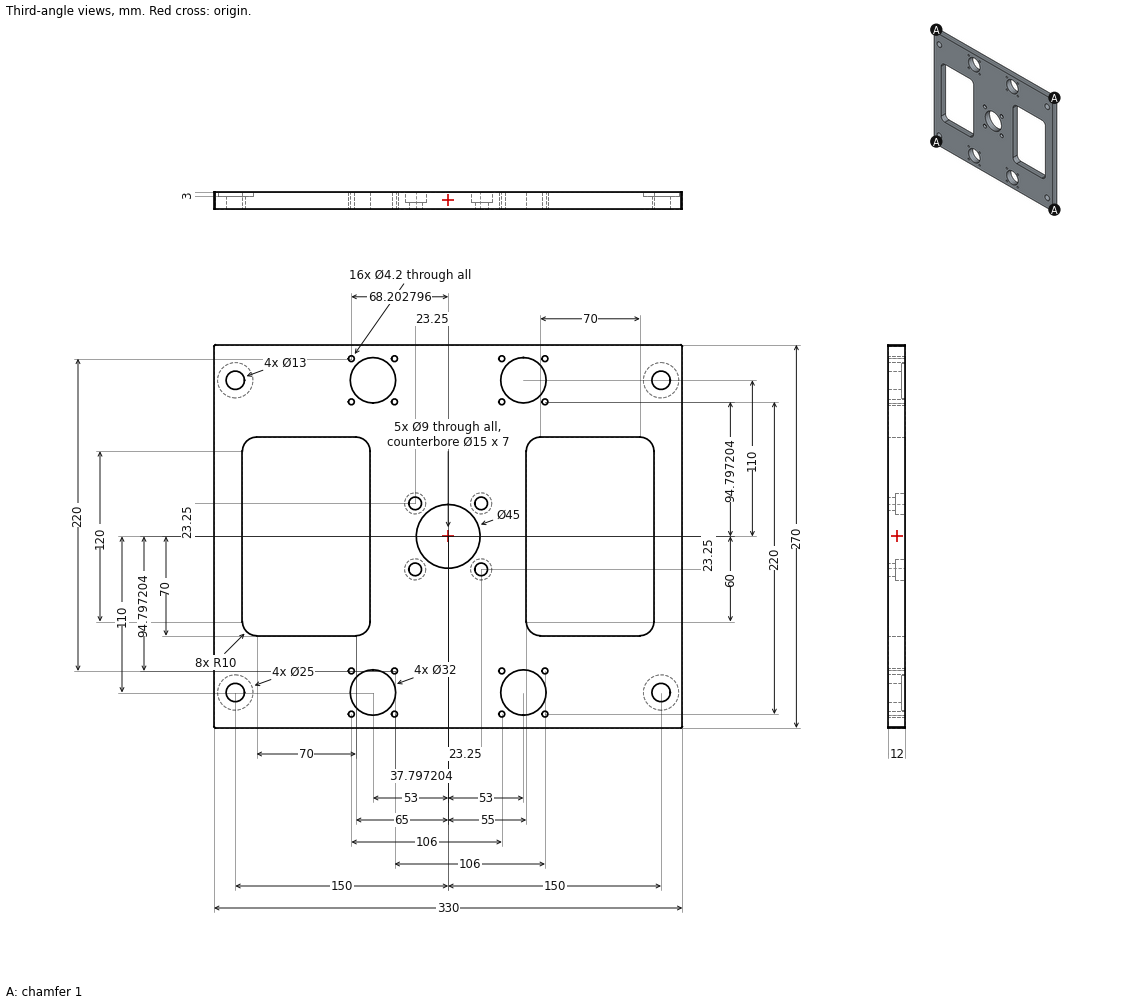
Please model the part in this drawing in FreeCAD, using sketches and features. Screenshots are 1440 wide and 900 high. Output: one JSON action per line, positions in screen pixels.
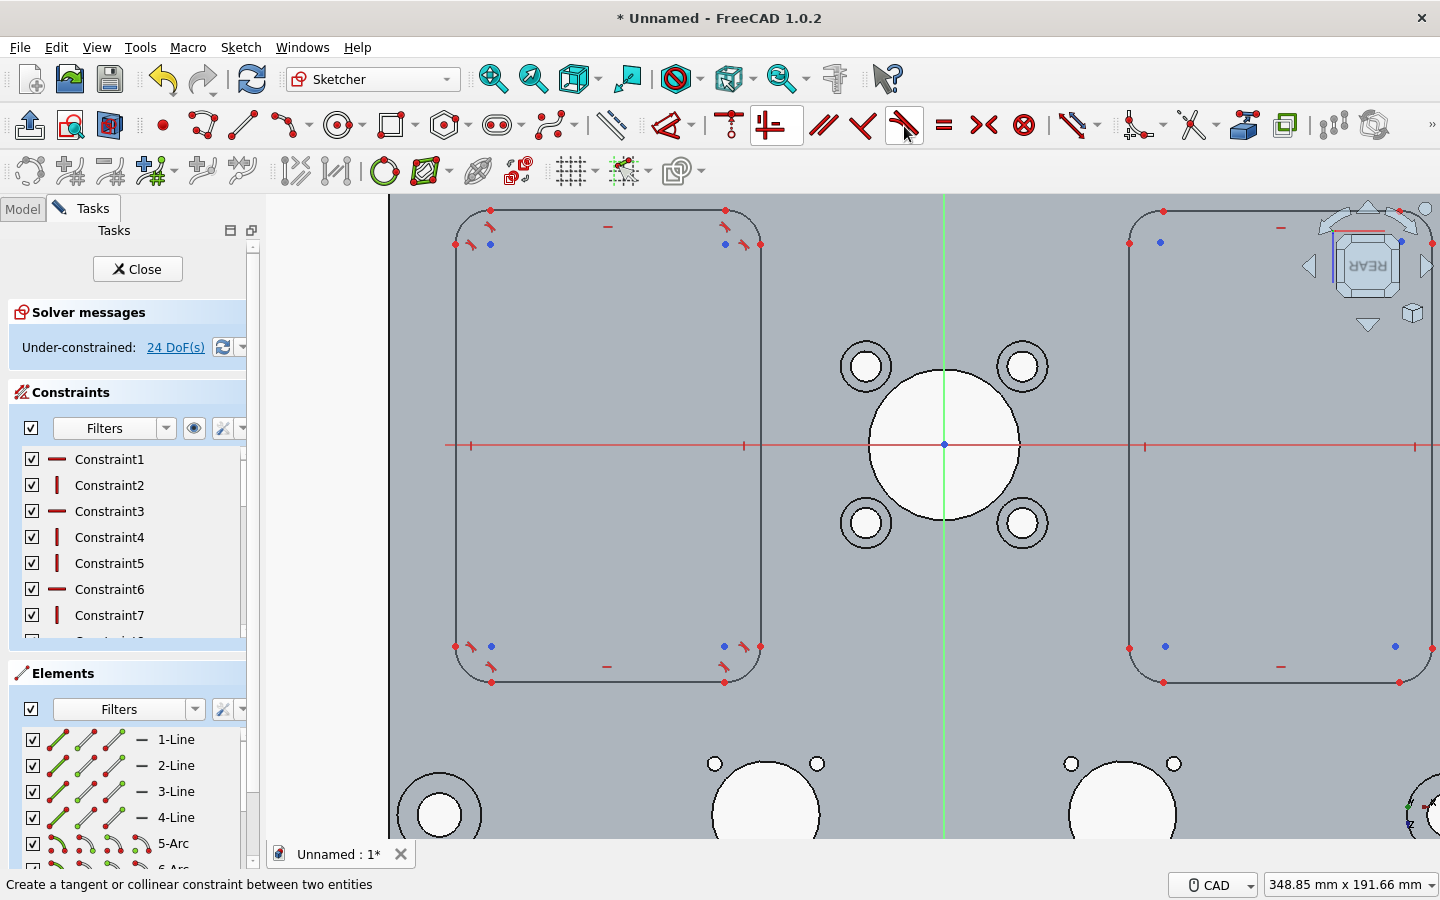
{"action": "left_click", "coordinate": [1129, 365]}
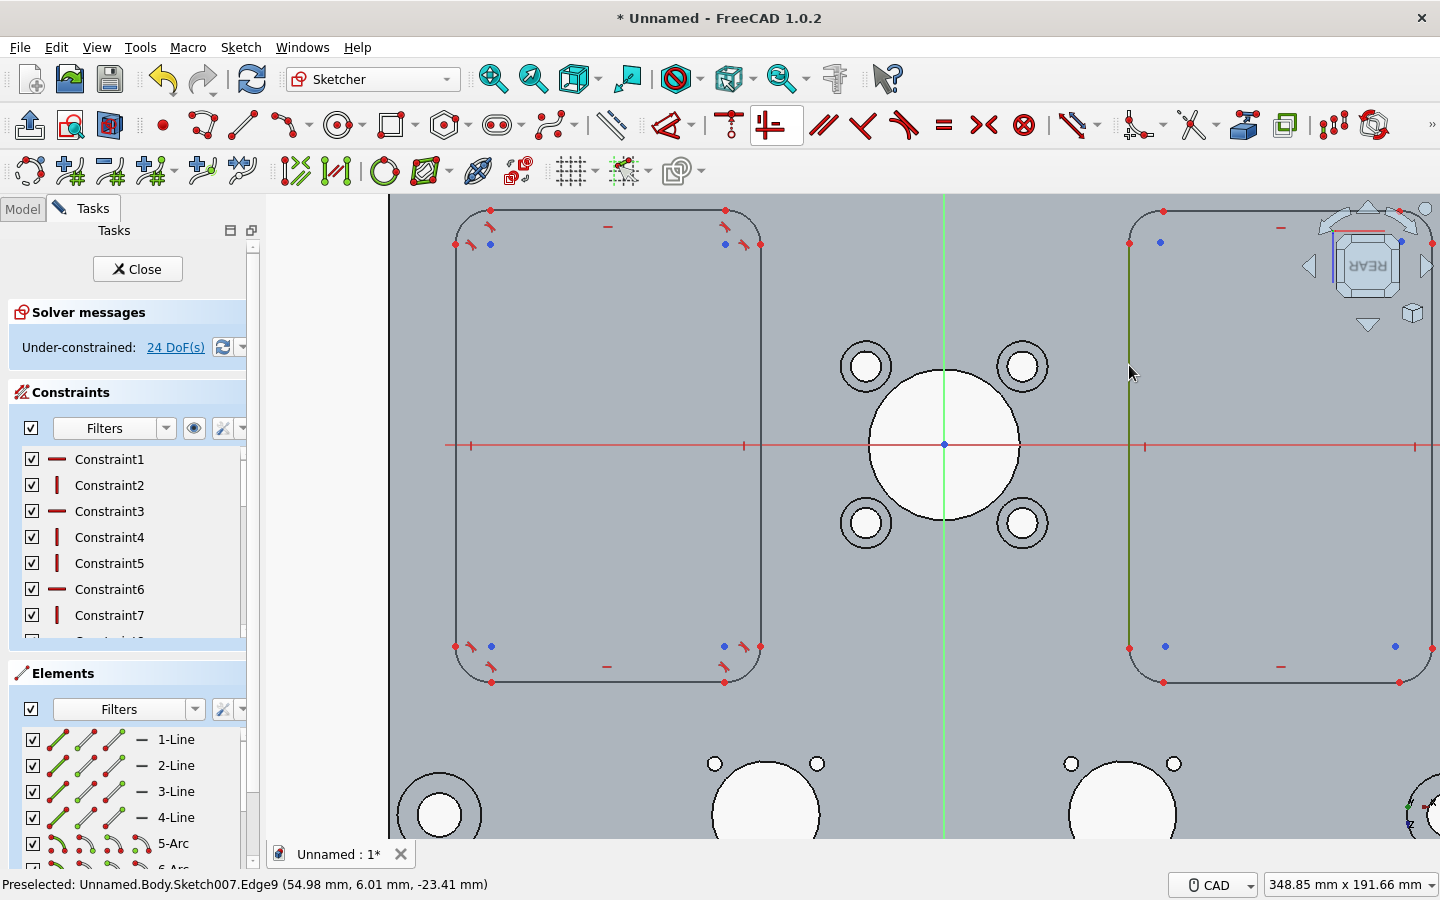
{"action": "left_click", "coordinate": [1133, 663]}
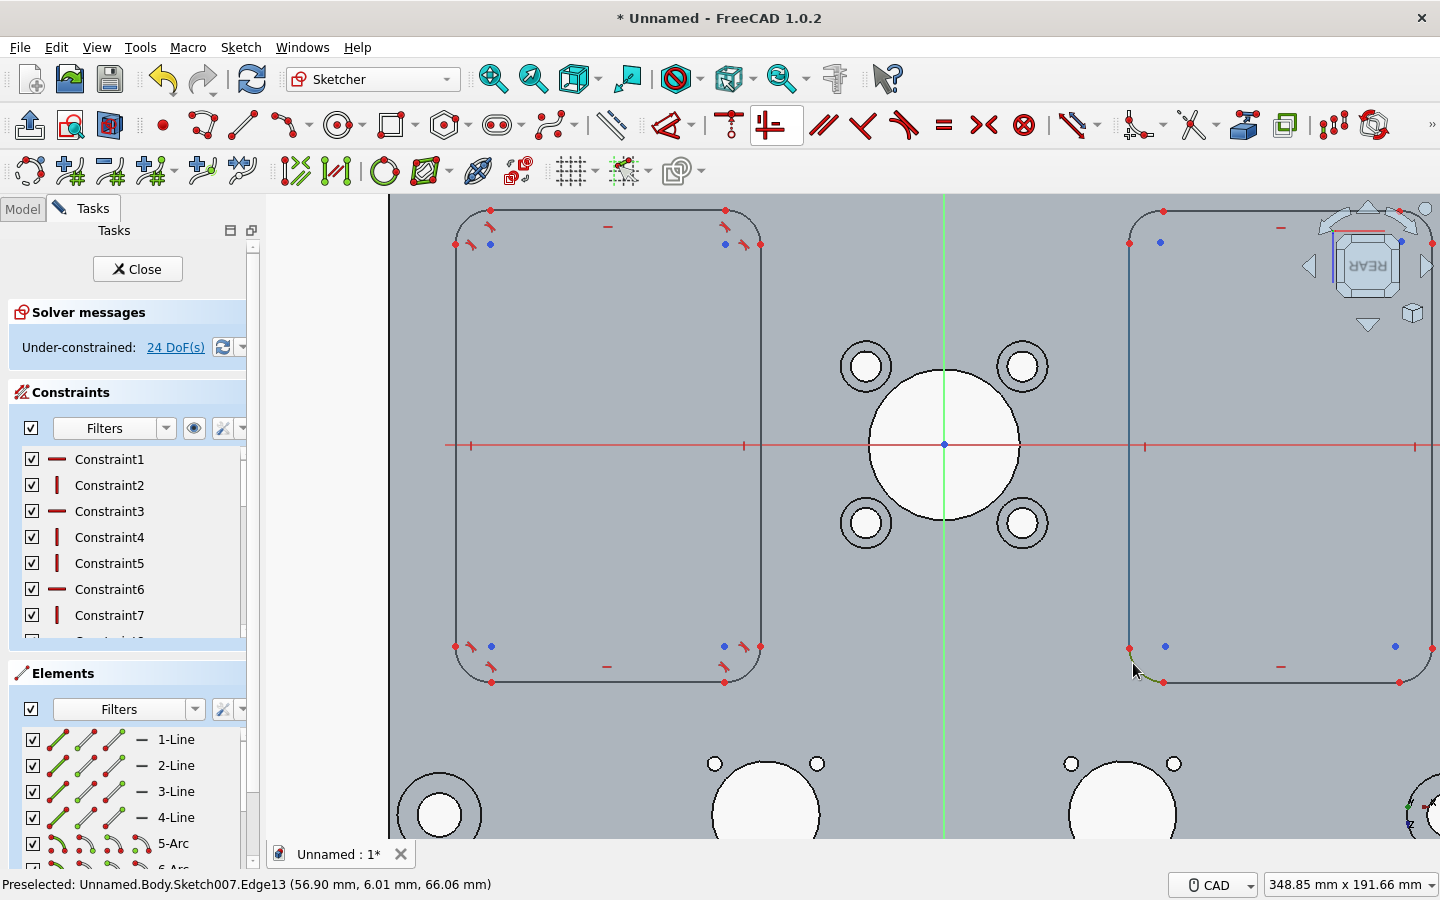
{"action": "left_click", "coordinate": [904, 126]}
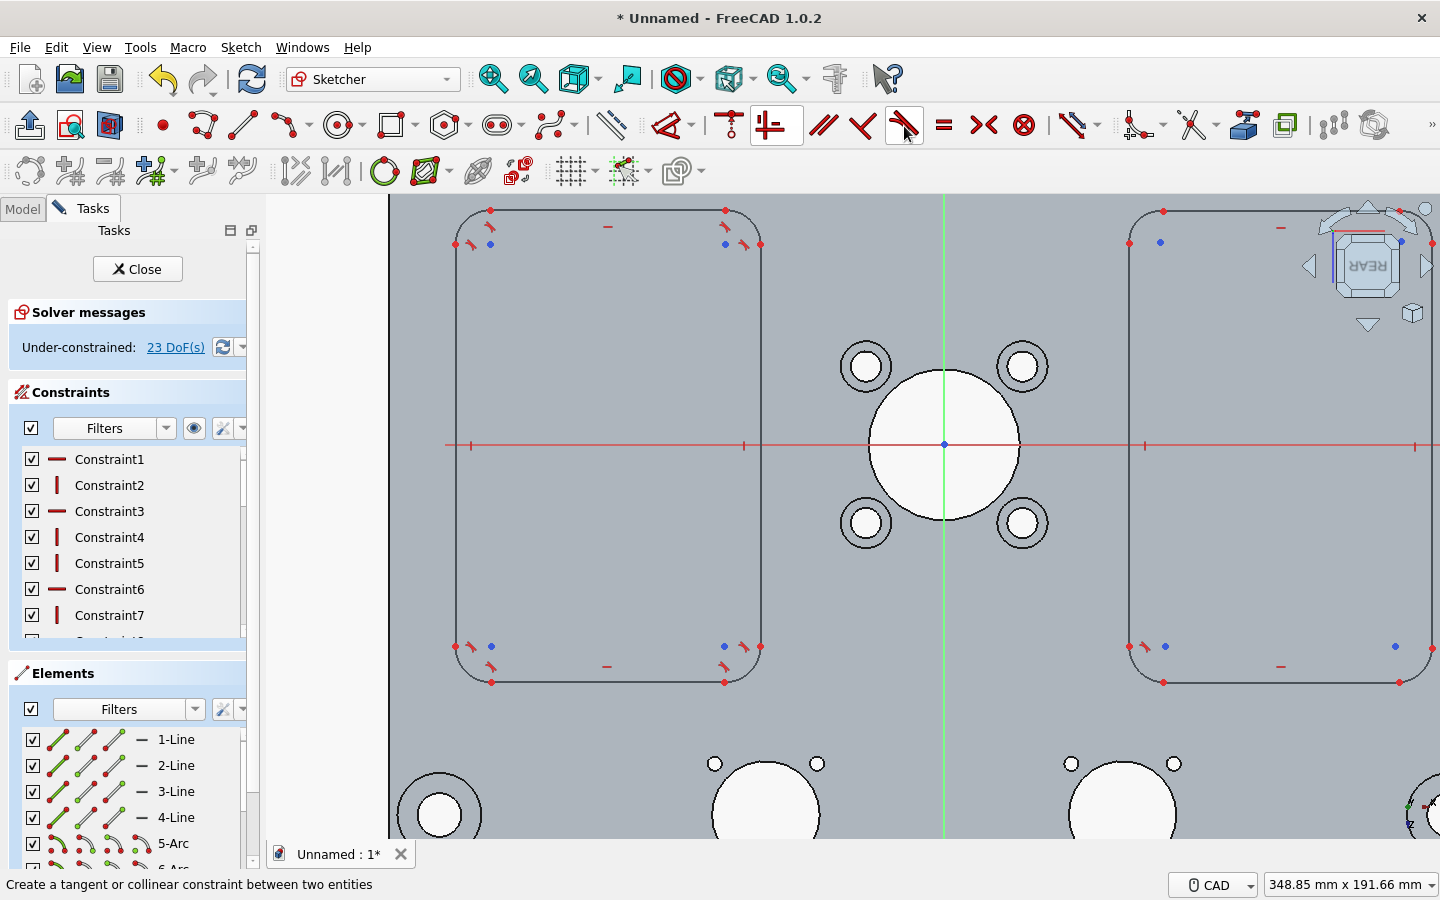
{"action": "left_click", "coordinate": [1129, 365]}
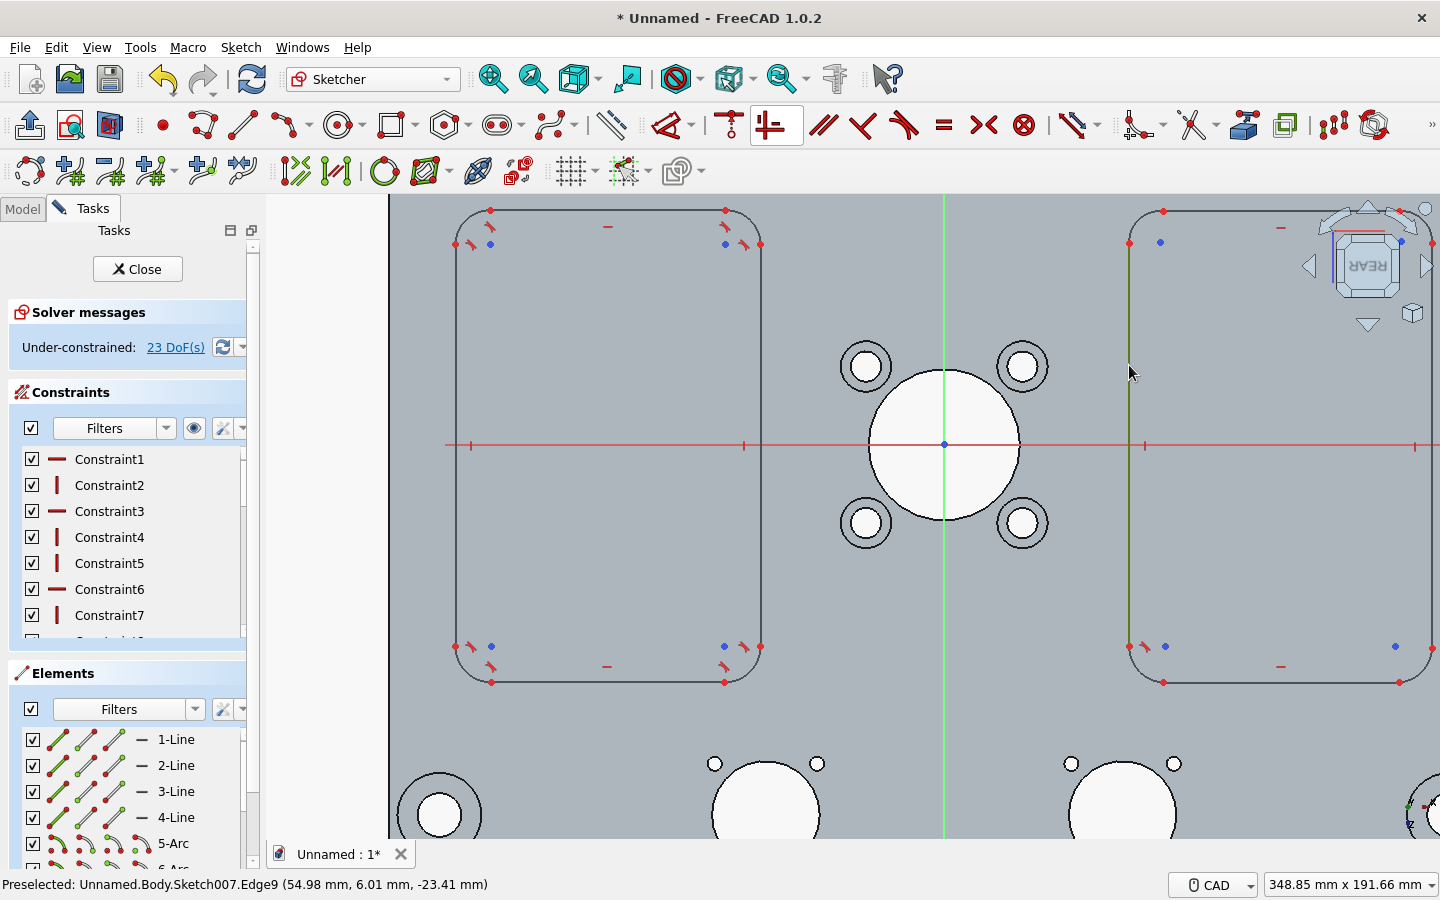
{"action": "left_click", "coordinate": [1132, 228]}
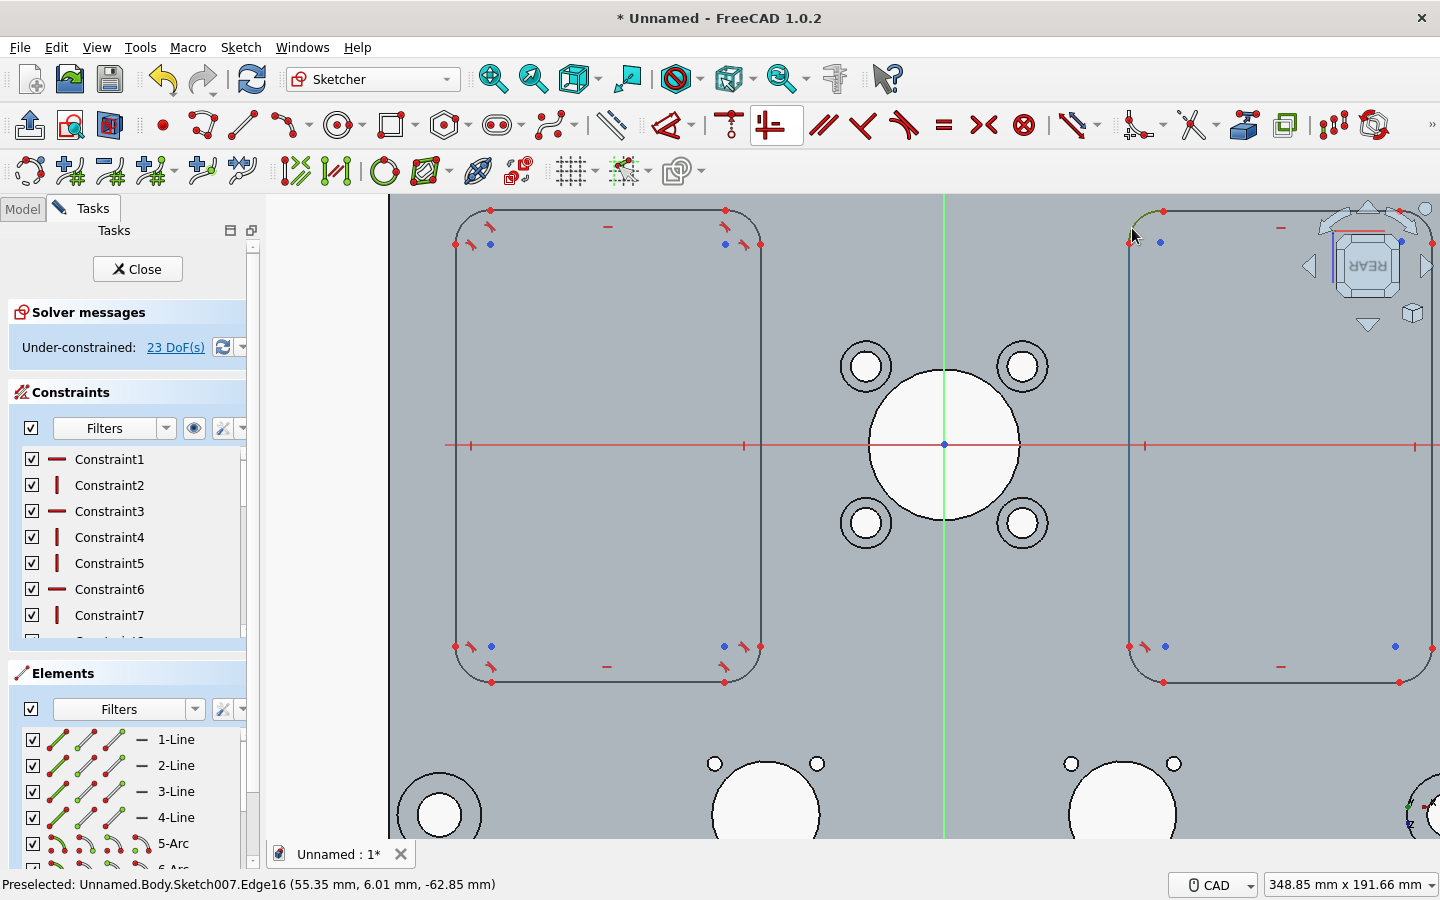
{"action": "left_click", "coordinate": [904, 126]}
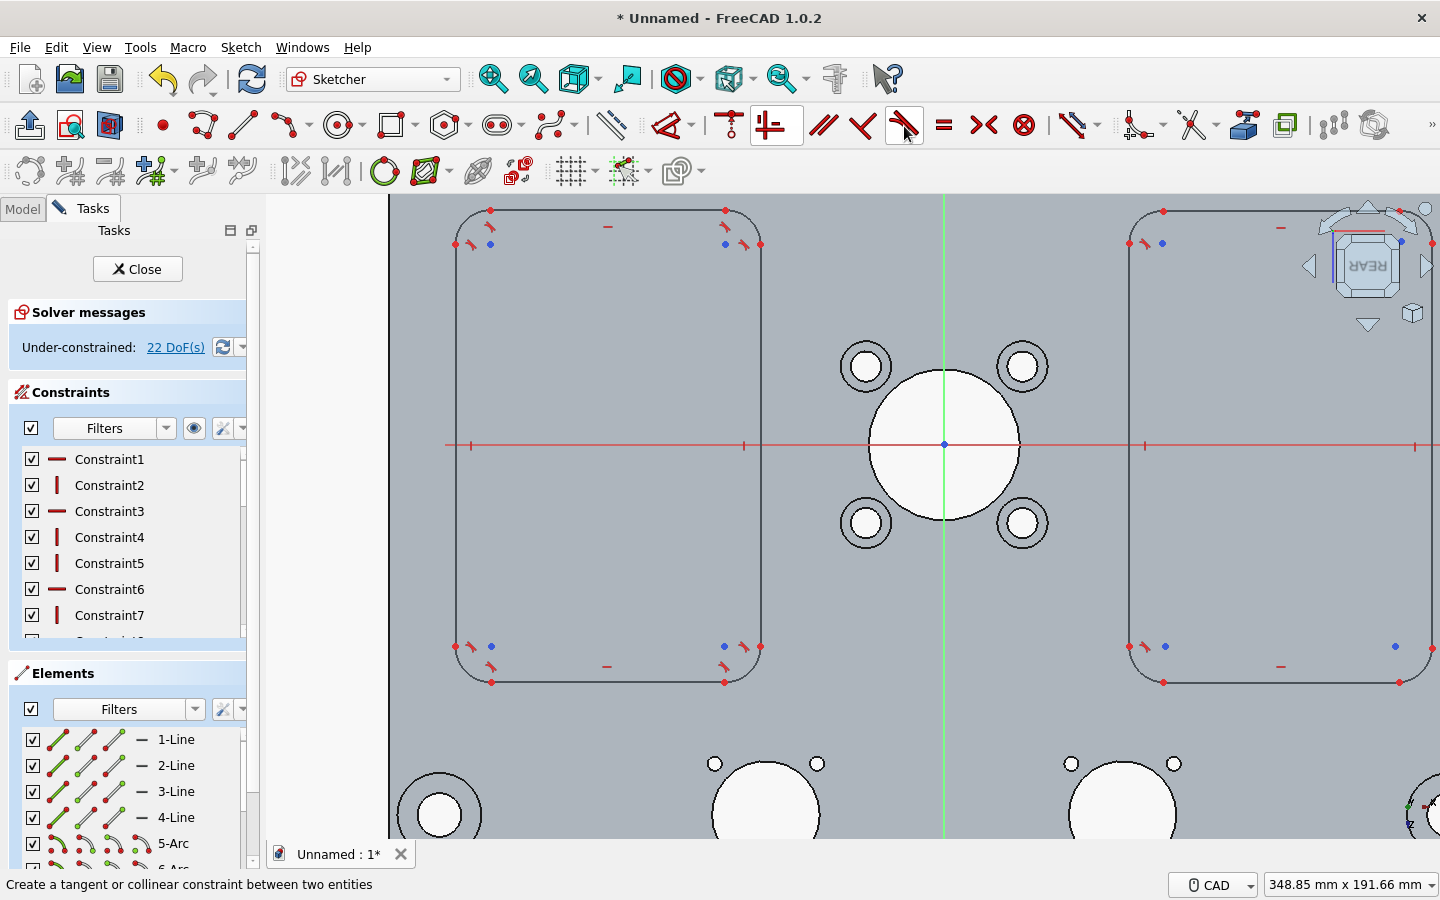
{"action": "left_click", "coordinate": [1234, 683]}